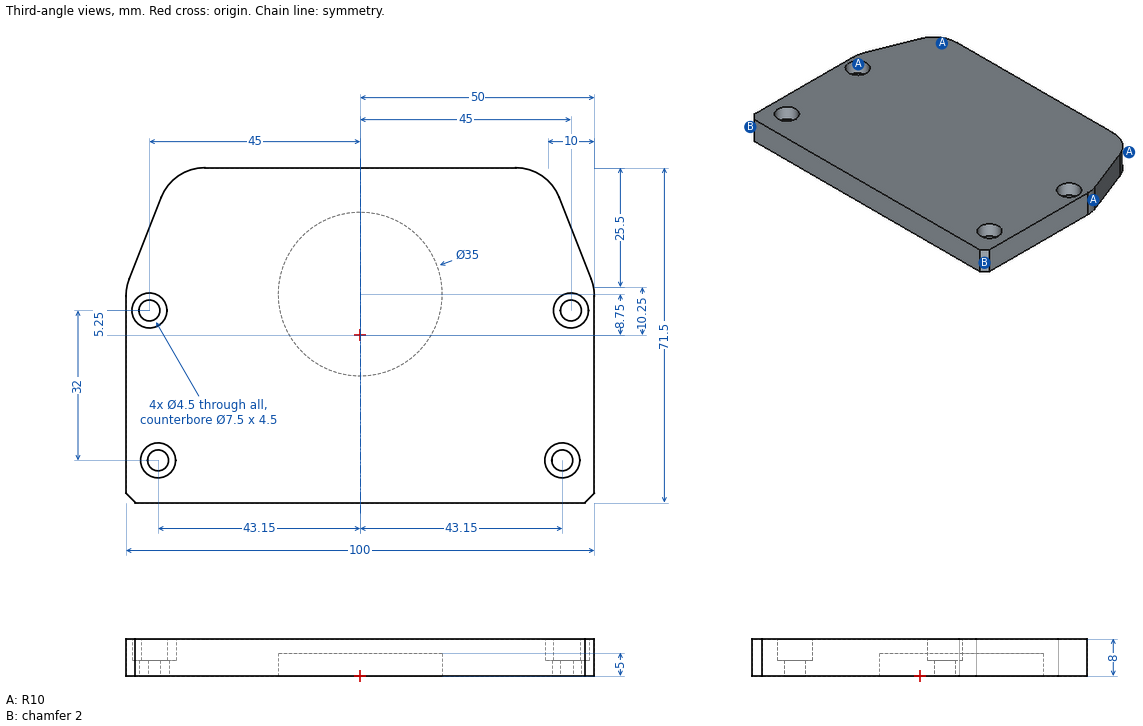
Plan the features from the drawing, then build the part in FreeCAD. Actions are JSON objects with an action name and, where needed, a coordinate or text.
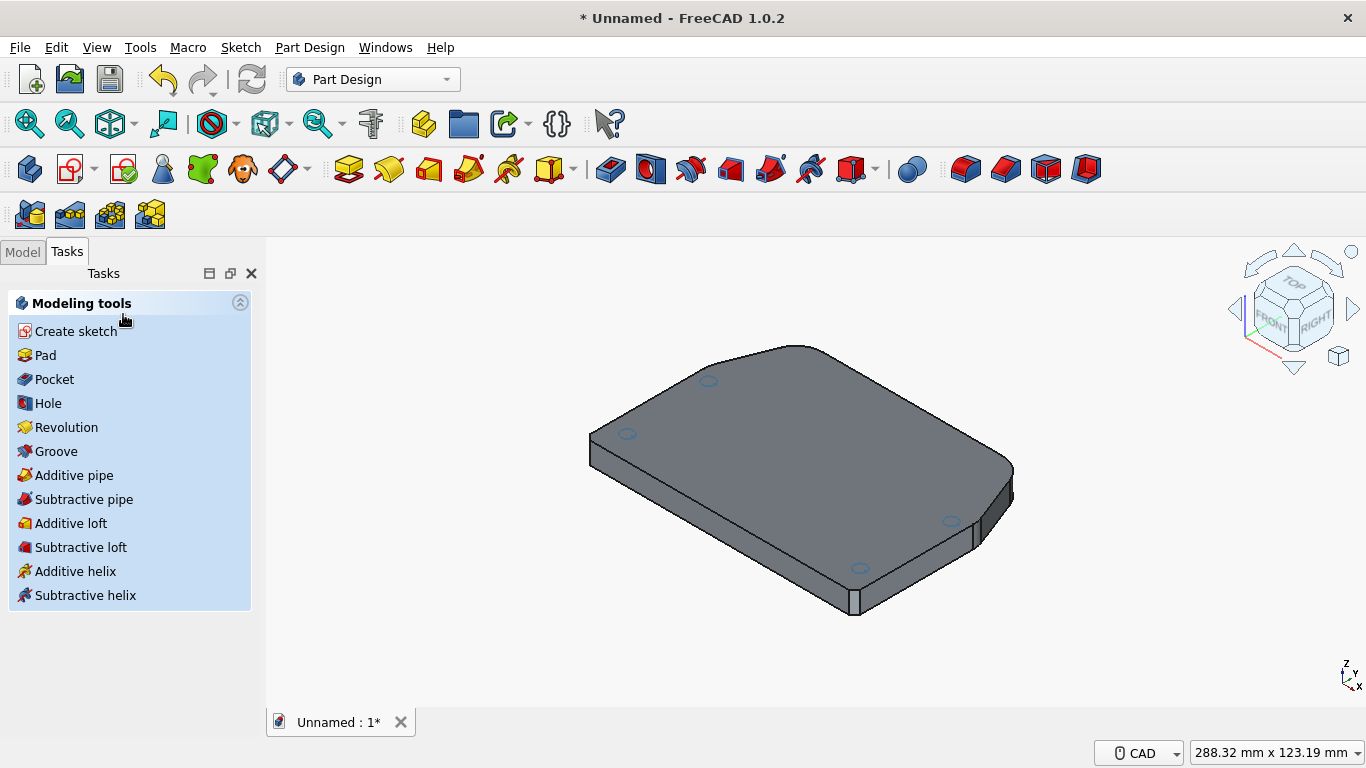
{"action": "left_click", "coordinate": [652, 170]}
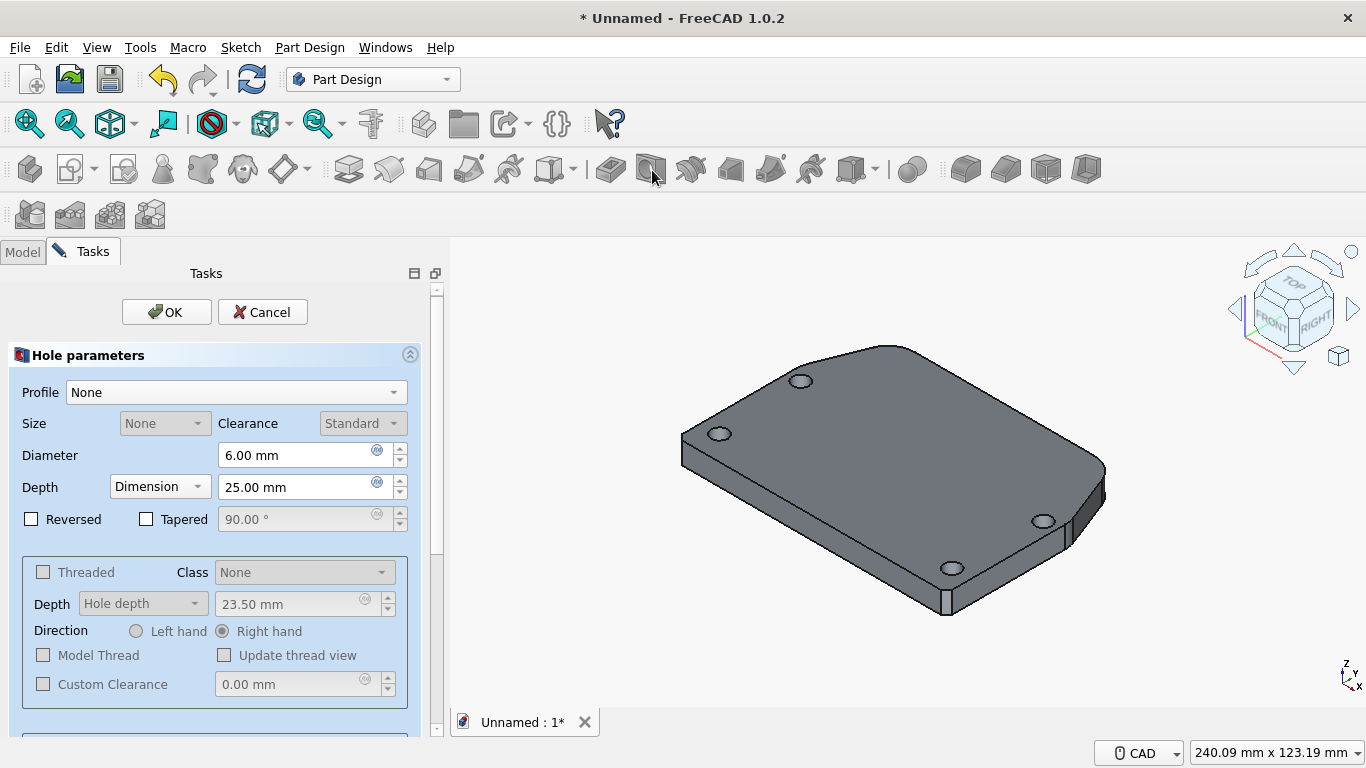
{"action": "triple_click", "coordinate": [305, 455]}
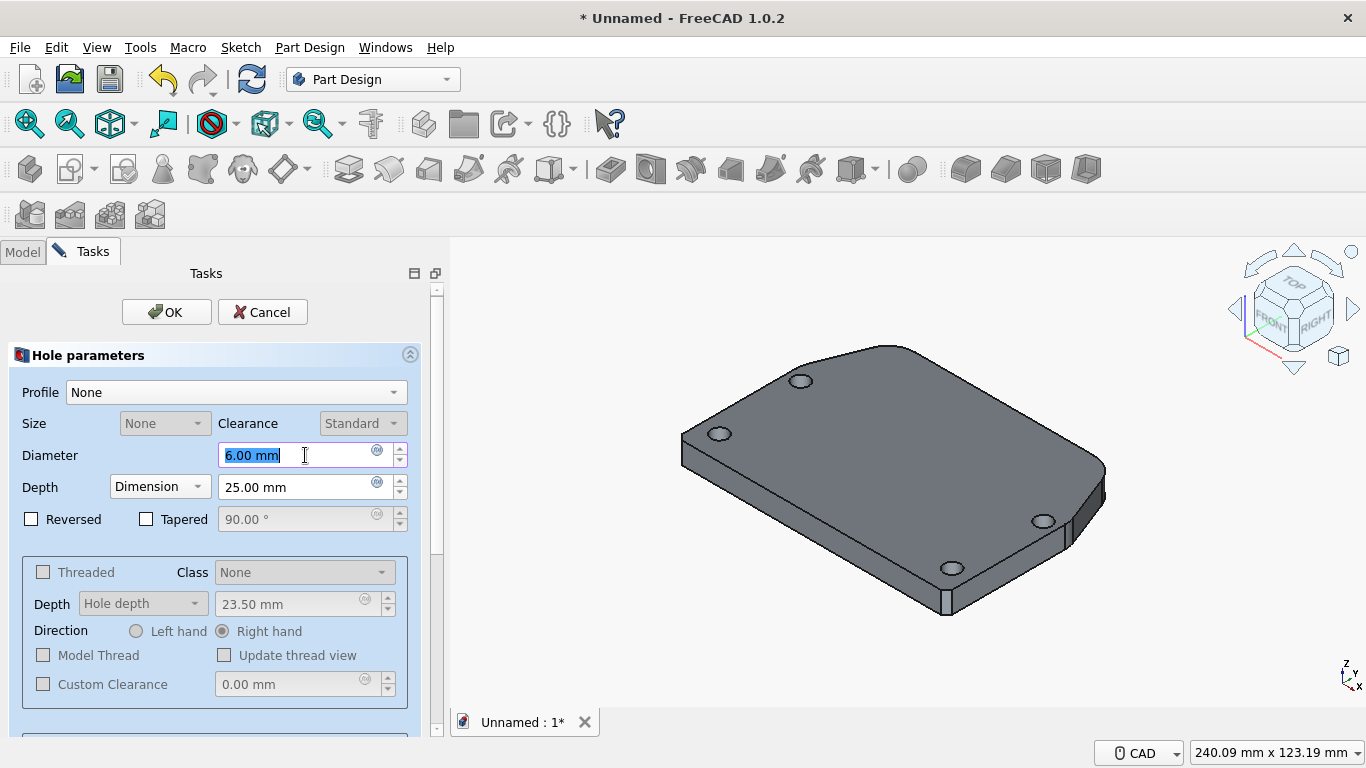
{"action": "type", "text": "4.5"}
{"action": "key", "text": "Tab"}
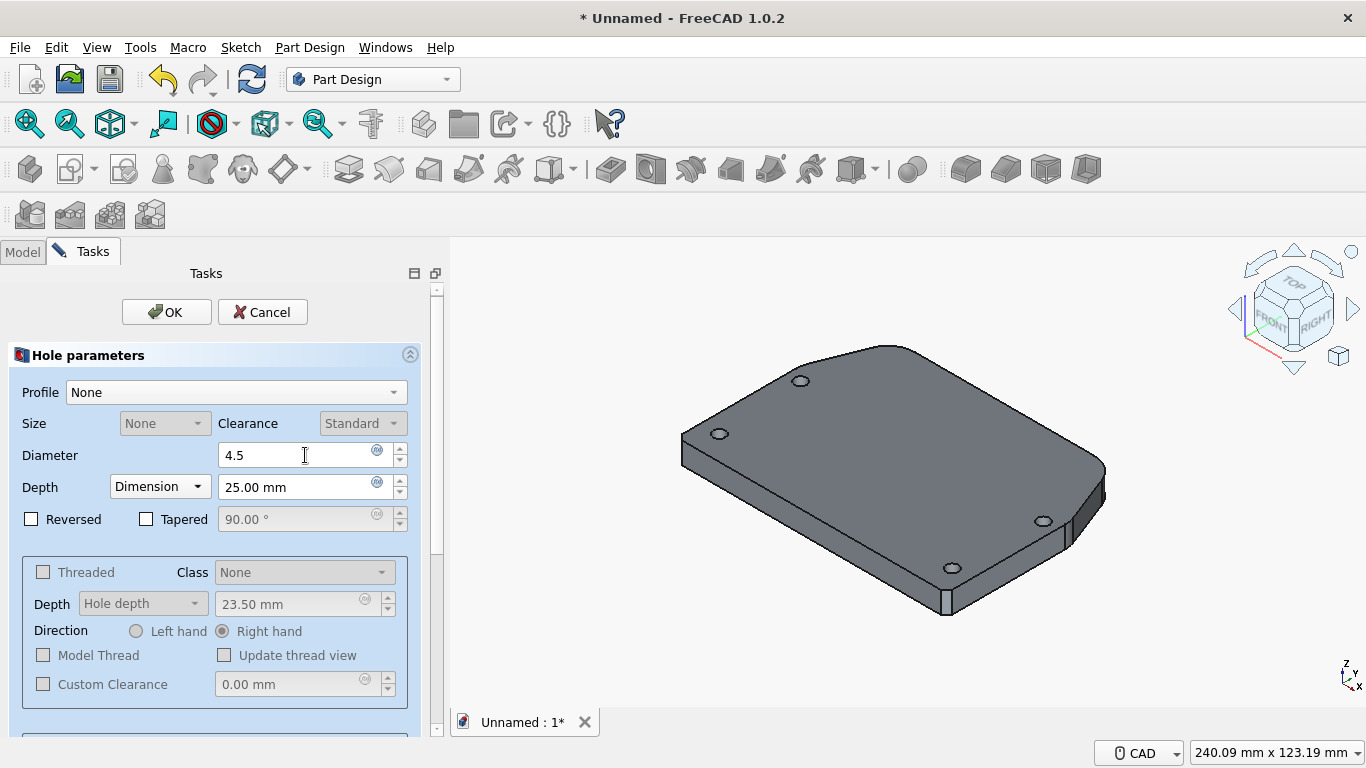
{"action": "left_click", "coordinate": [161, 486]}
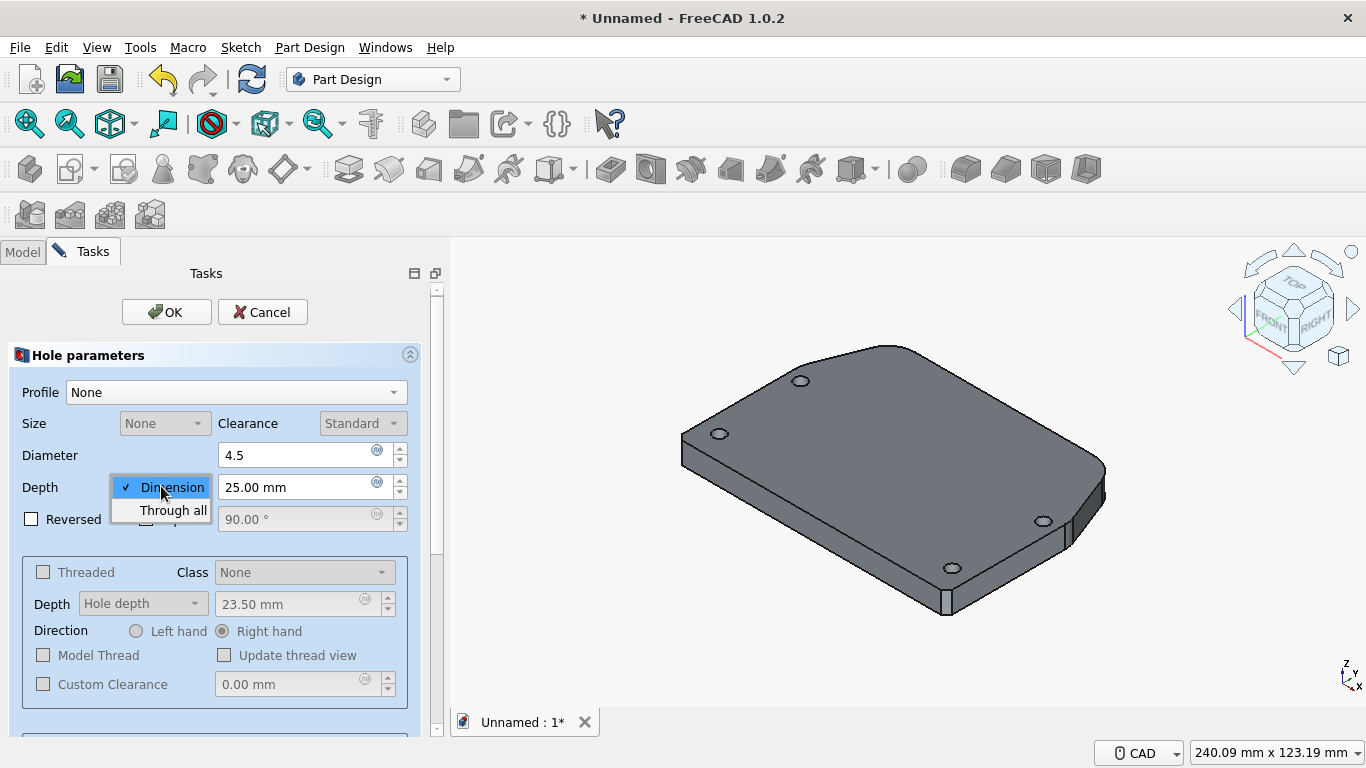
{"action": "left_click", "coordinate": [160, 510]}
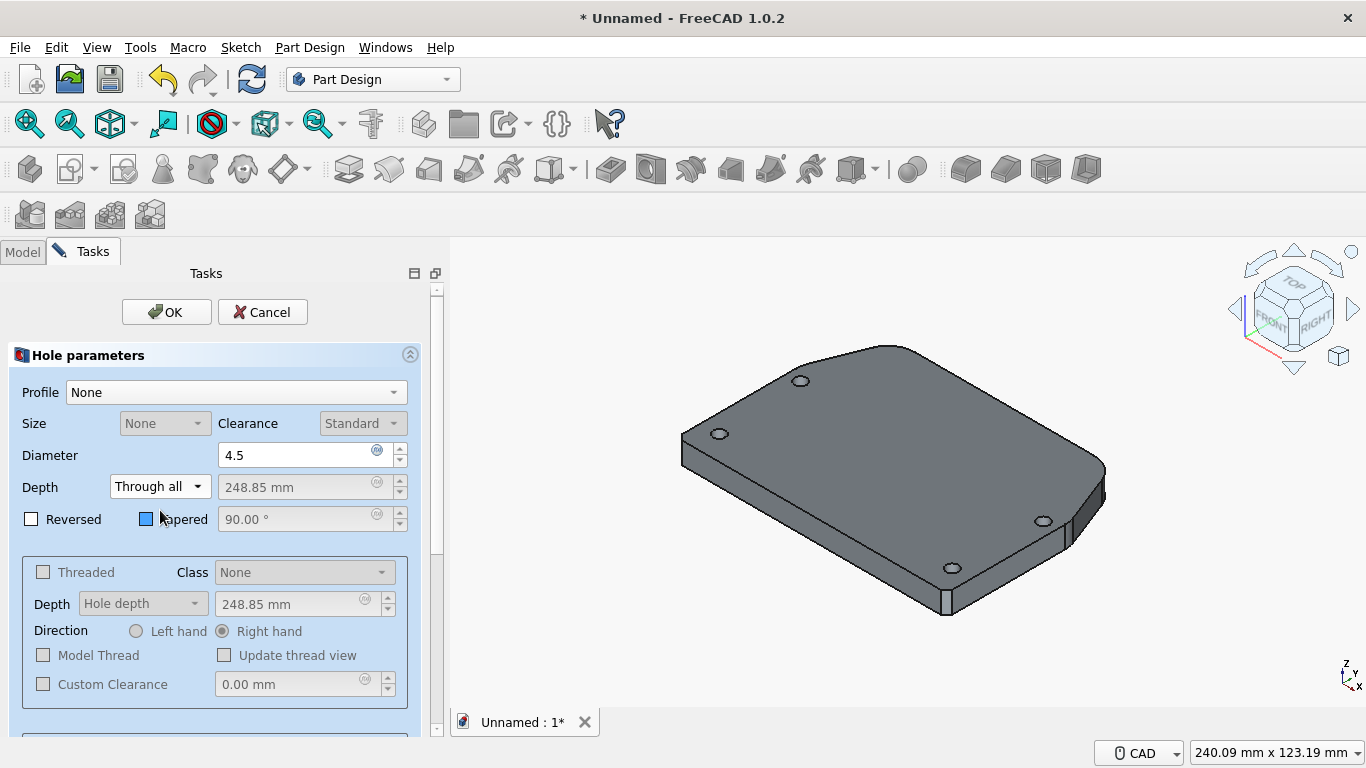
{"action": "scroll", "coordinate": [437, 510], "scroll_direction": "down", "scroll_amount": 2}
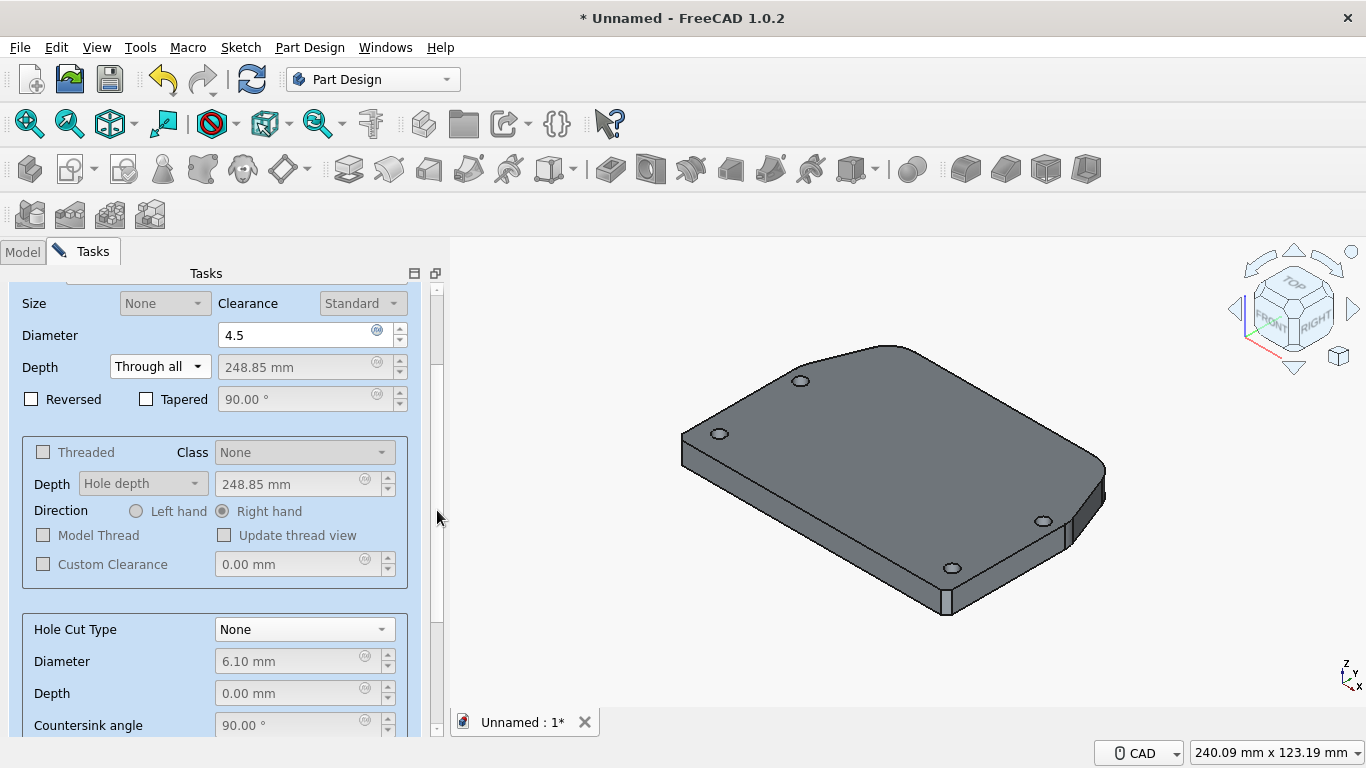
{"action": "left_click", "coordinate": [306, 630]}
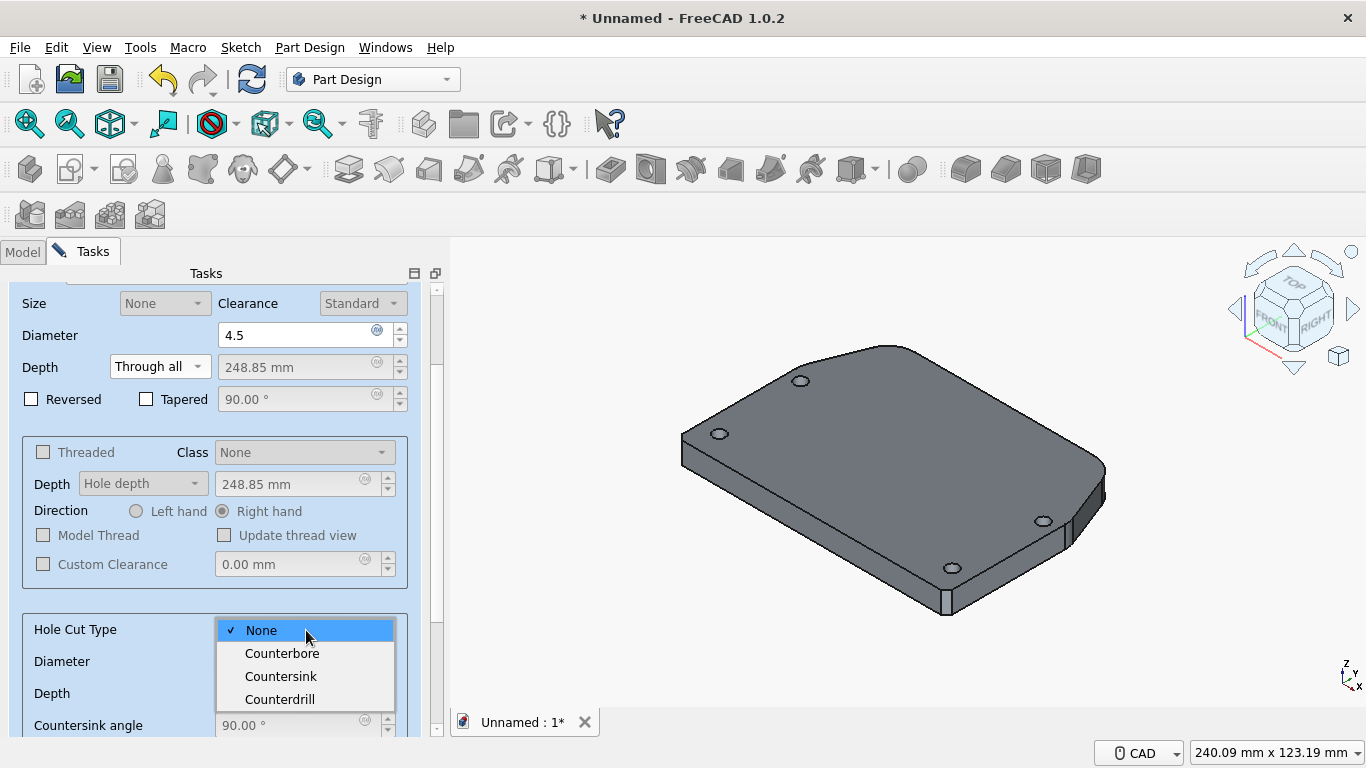
{"action": "left_click", "coordinate": [304, 654]}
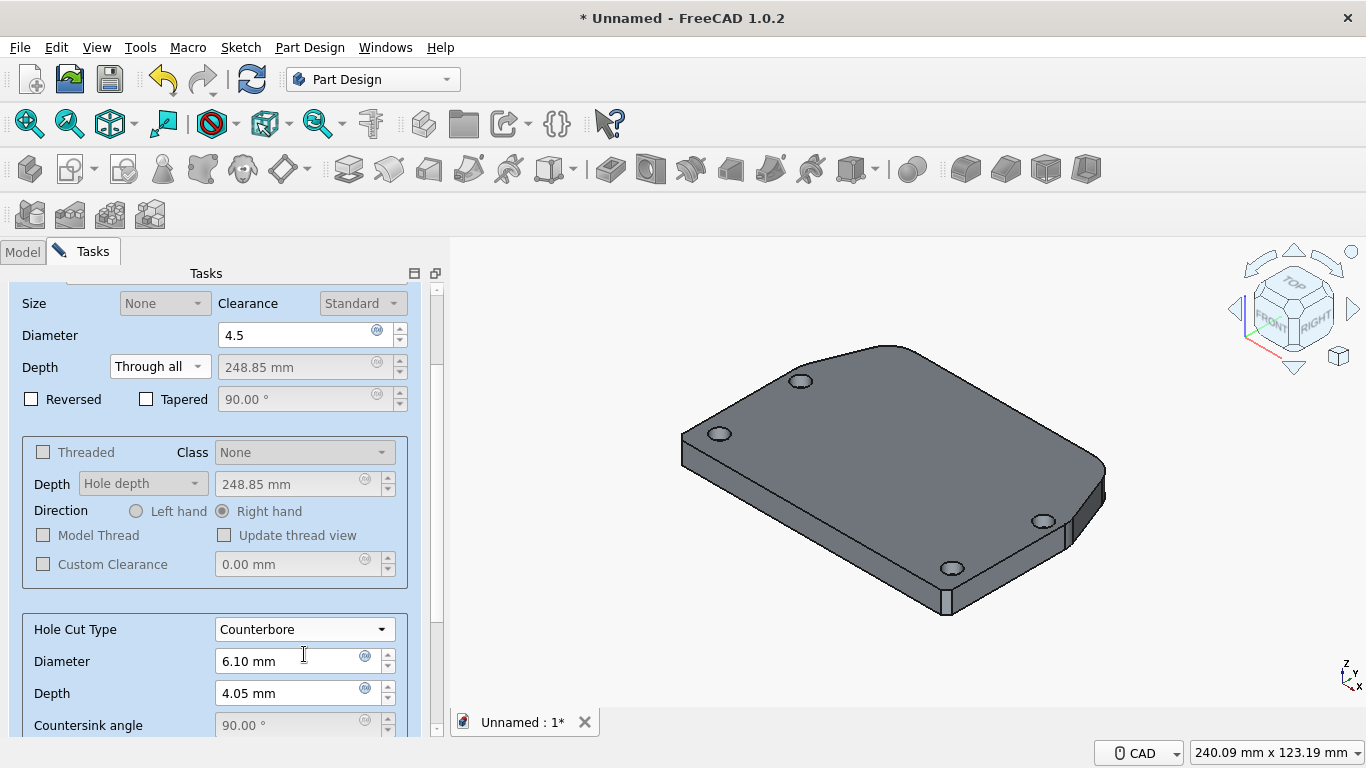
{"action": "triple_click", "coordinate": [298, 661]}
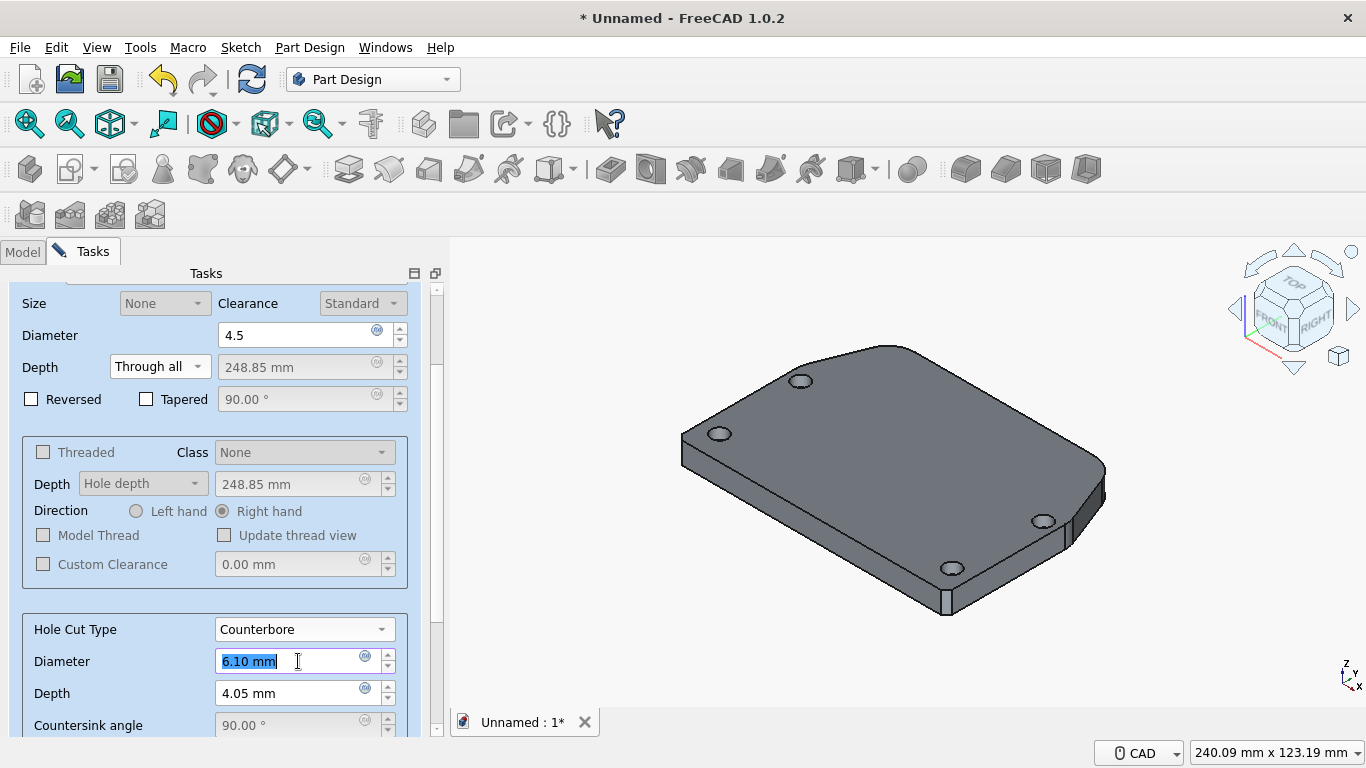
{"action": "type", "text": "7.5"}
{"action": "key", "text": "Tab"}